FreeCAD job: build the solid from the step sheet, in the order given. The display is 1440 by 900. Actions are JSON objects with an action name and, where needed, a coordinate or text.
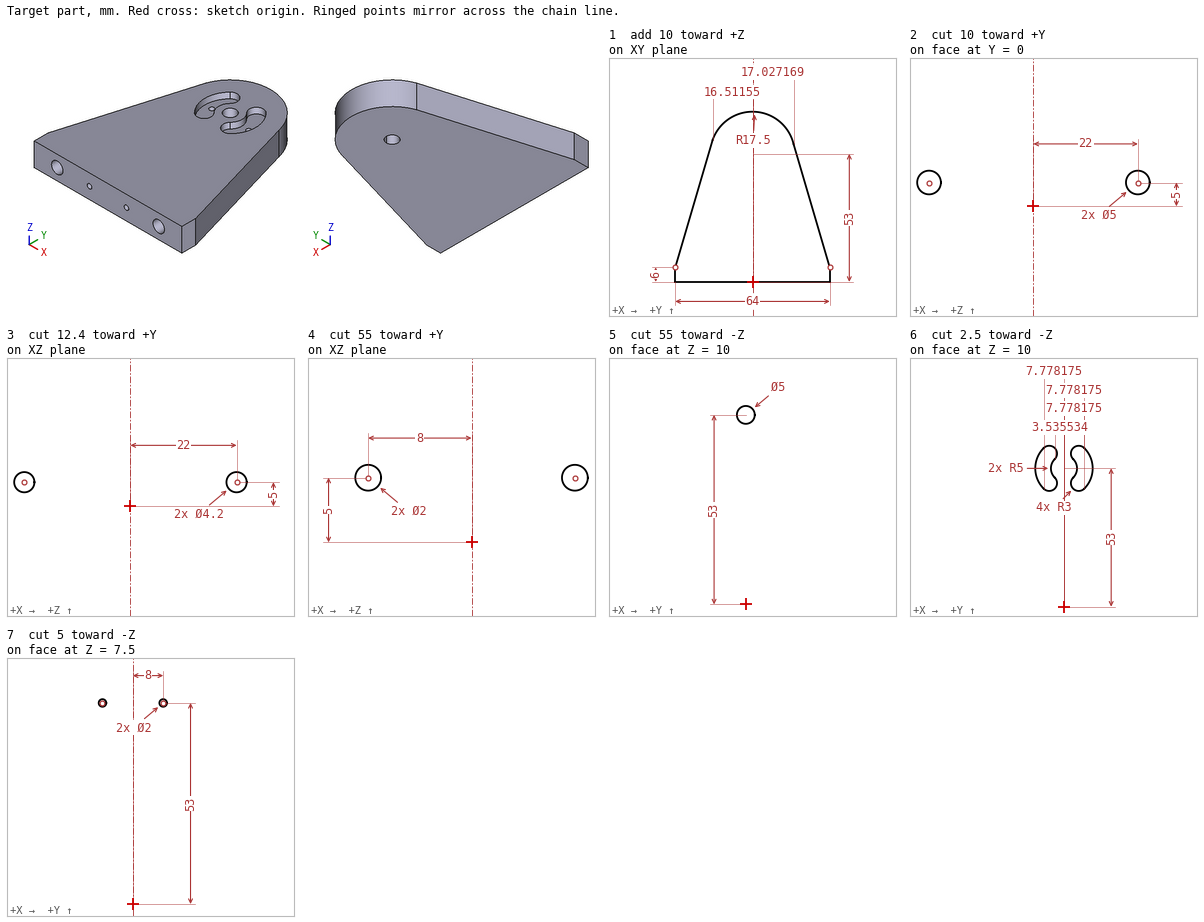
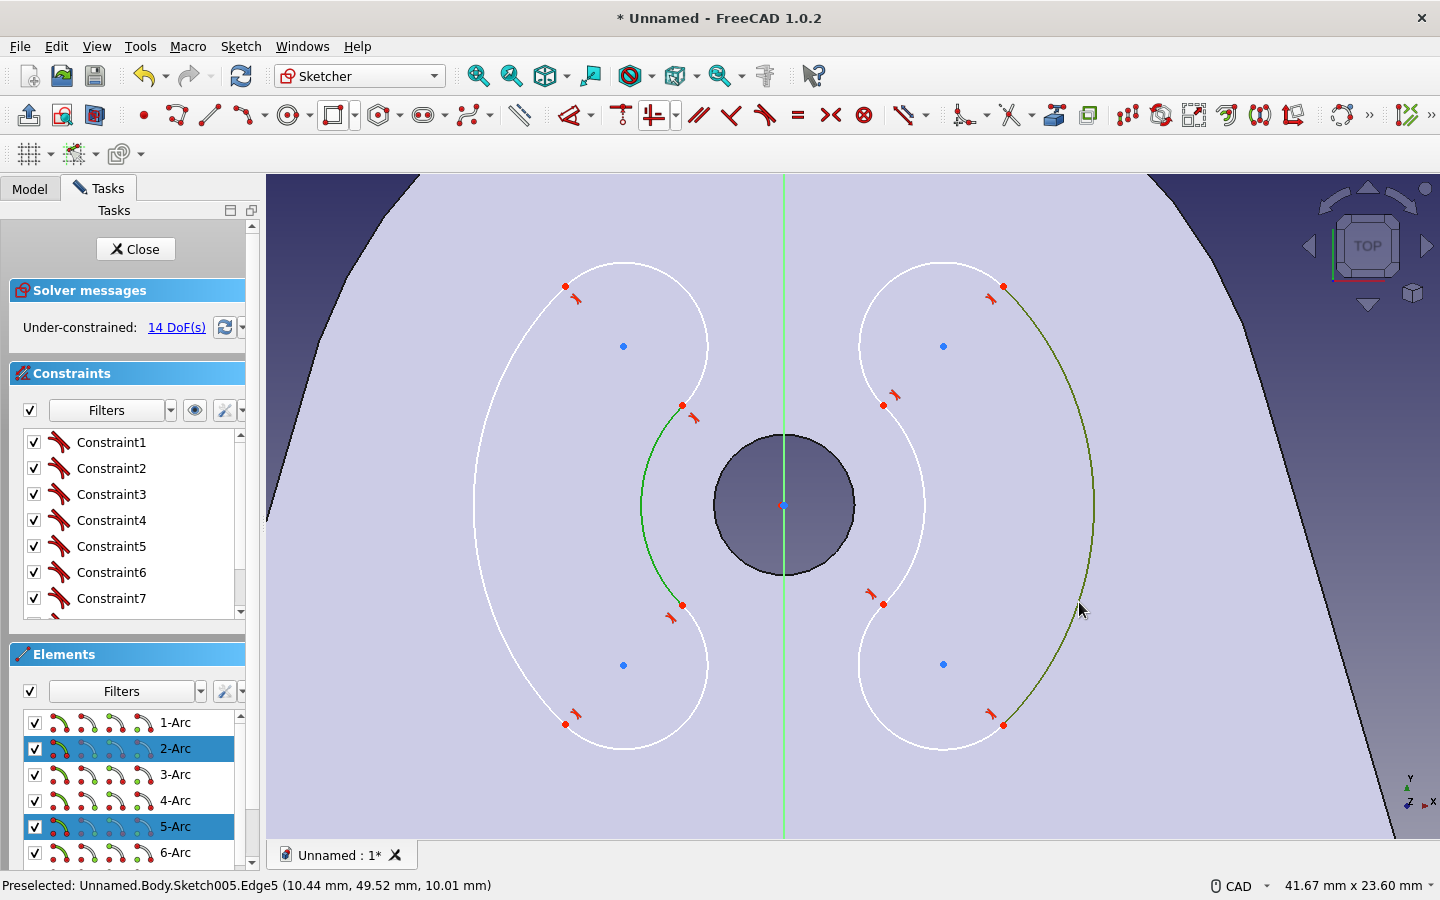
{"action": "left_click", "coordinate": [621, 116]}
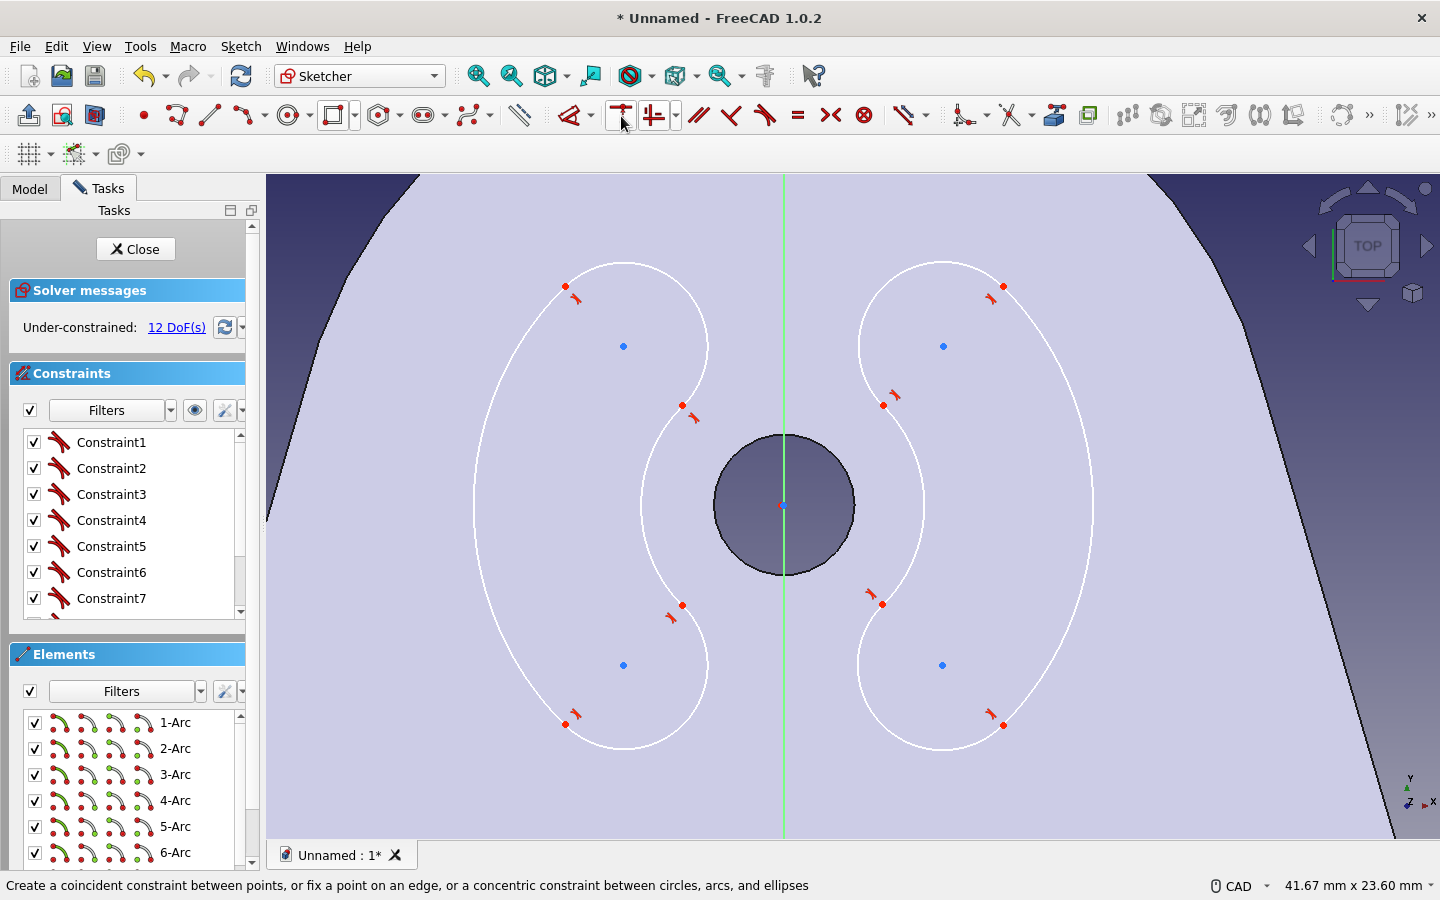
{"action": "left_click", "coordinate": [648, 462]}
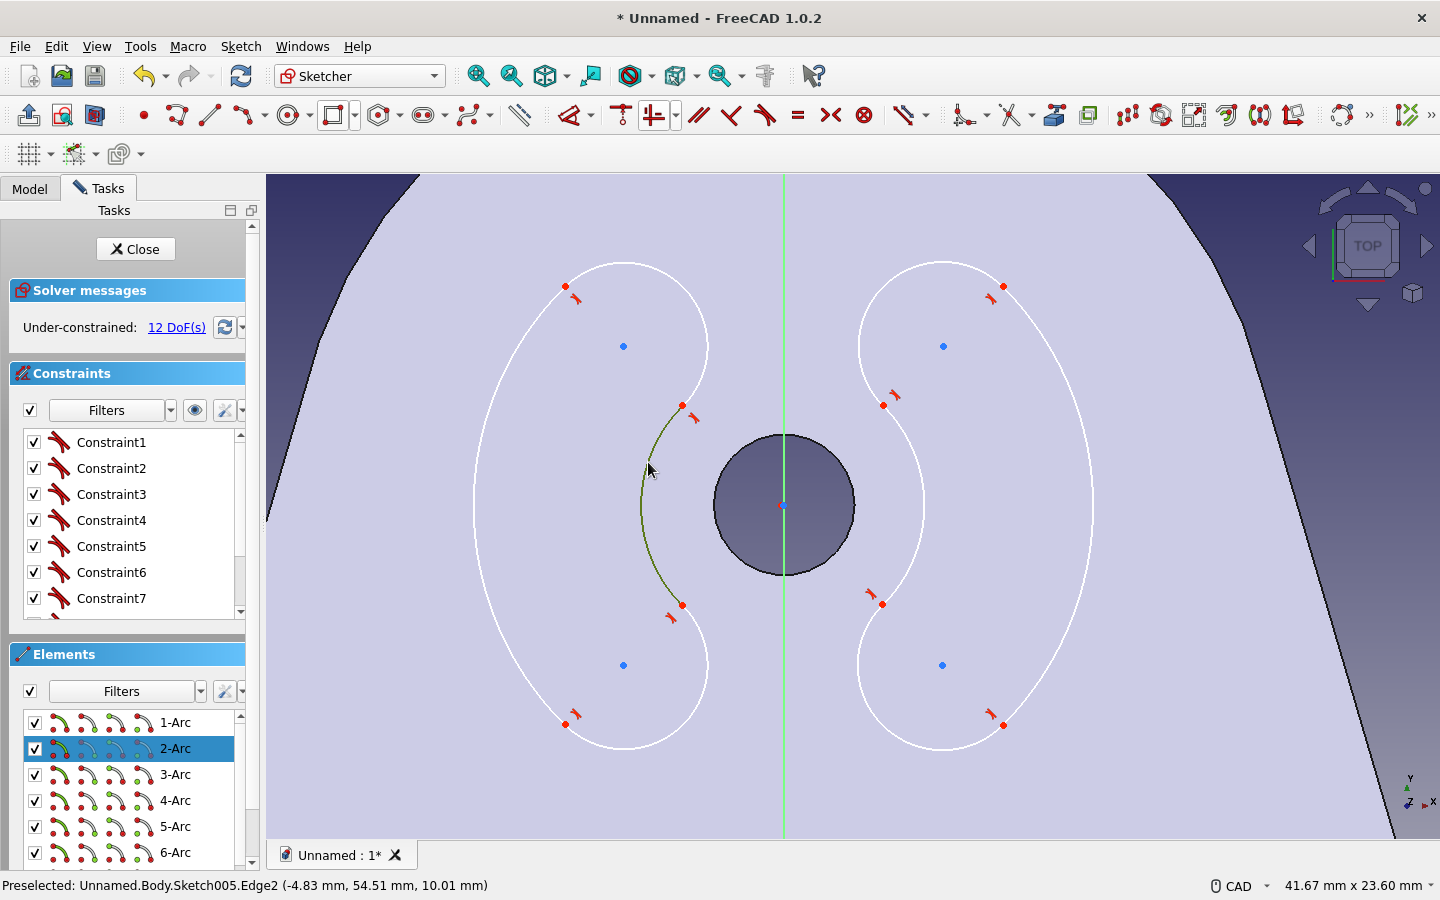
{"action": "left_click", "coordinate": [917, 549]}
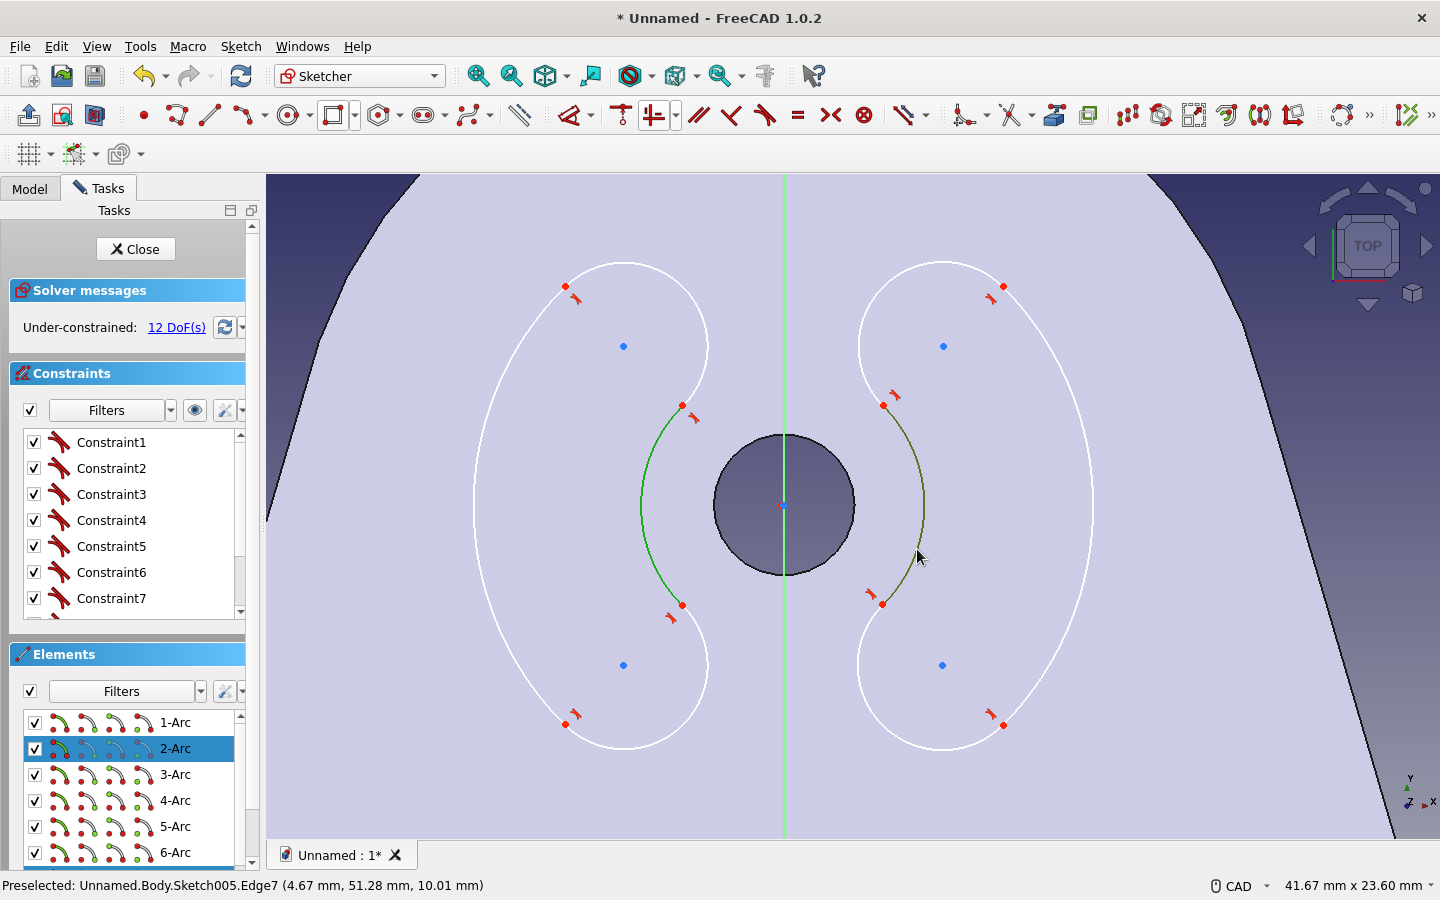
{"action": "left_click", "coordinate": [621, 116]}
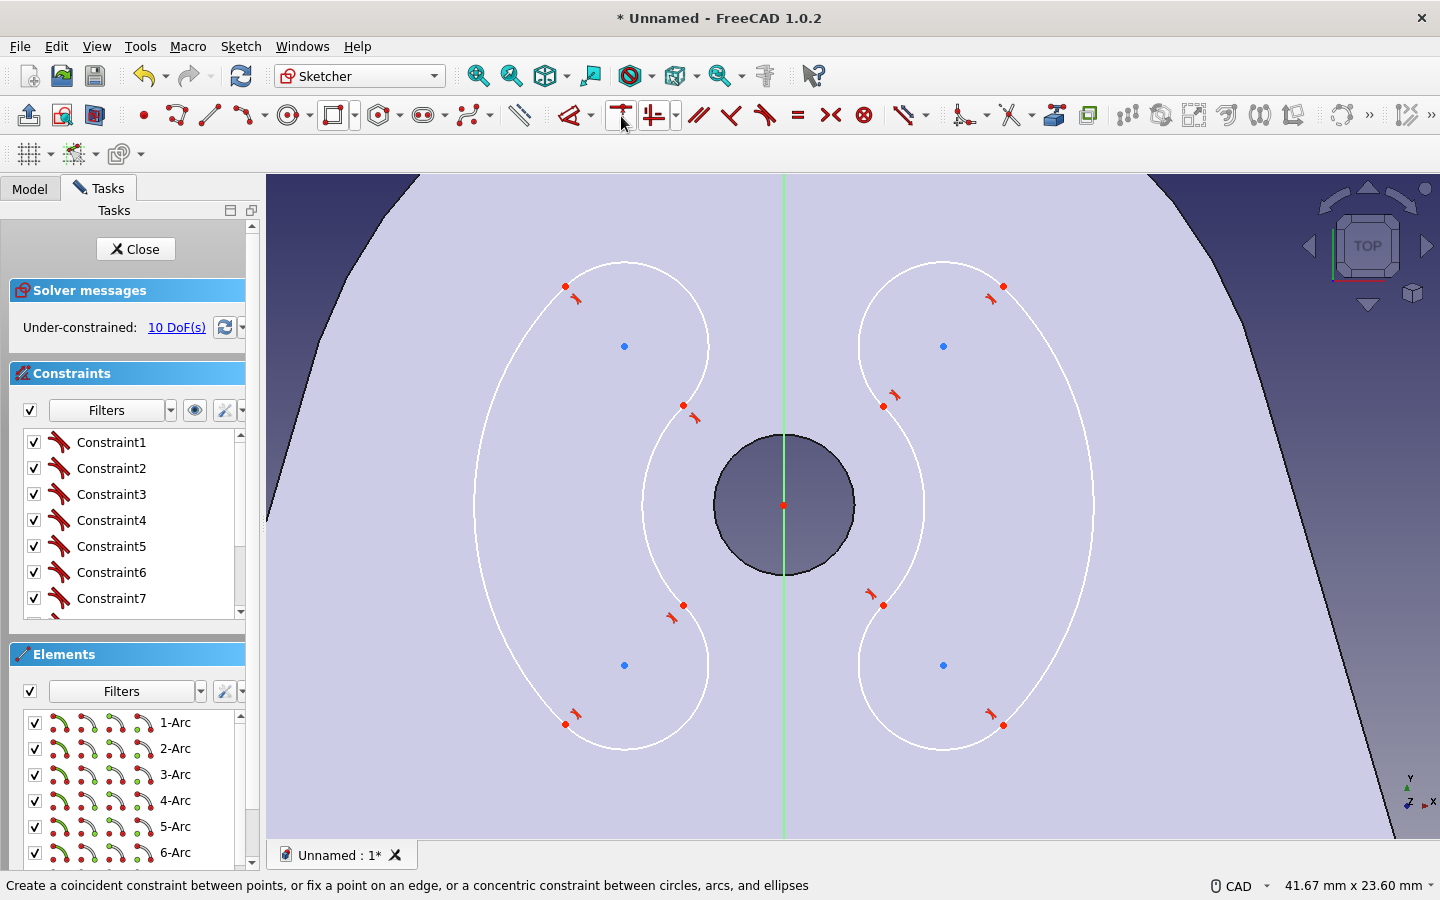
{"action": "left_click", "coordinate": [489, 410]}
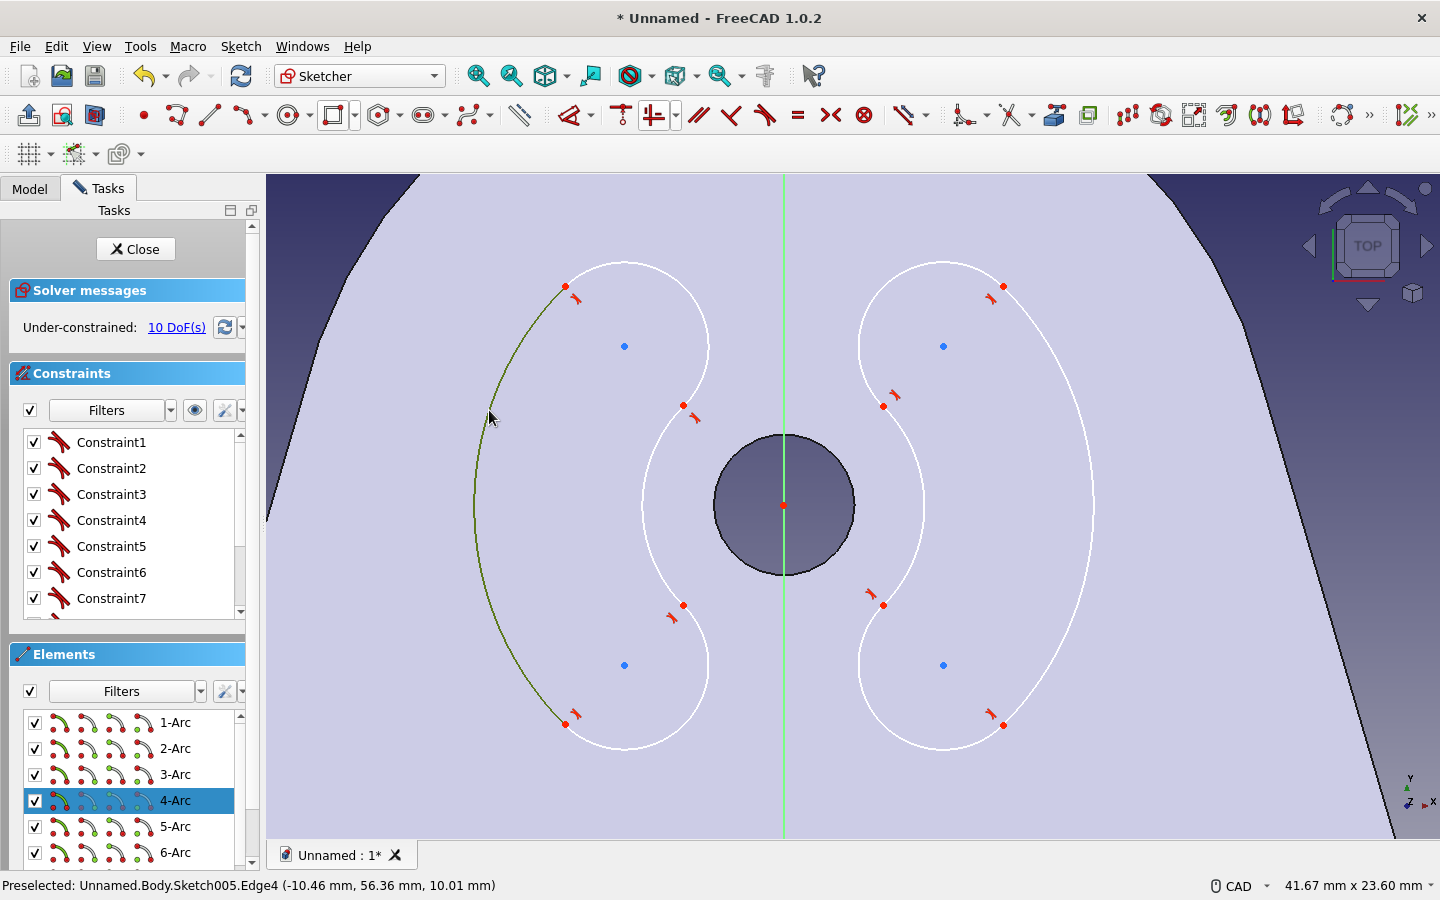
{"action": "left_click", "coordinate": [1078, 602]}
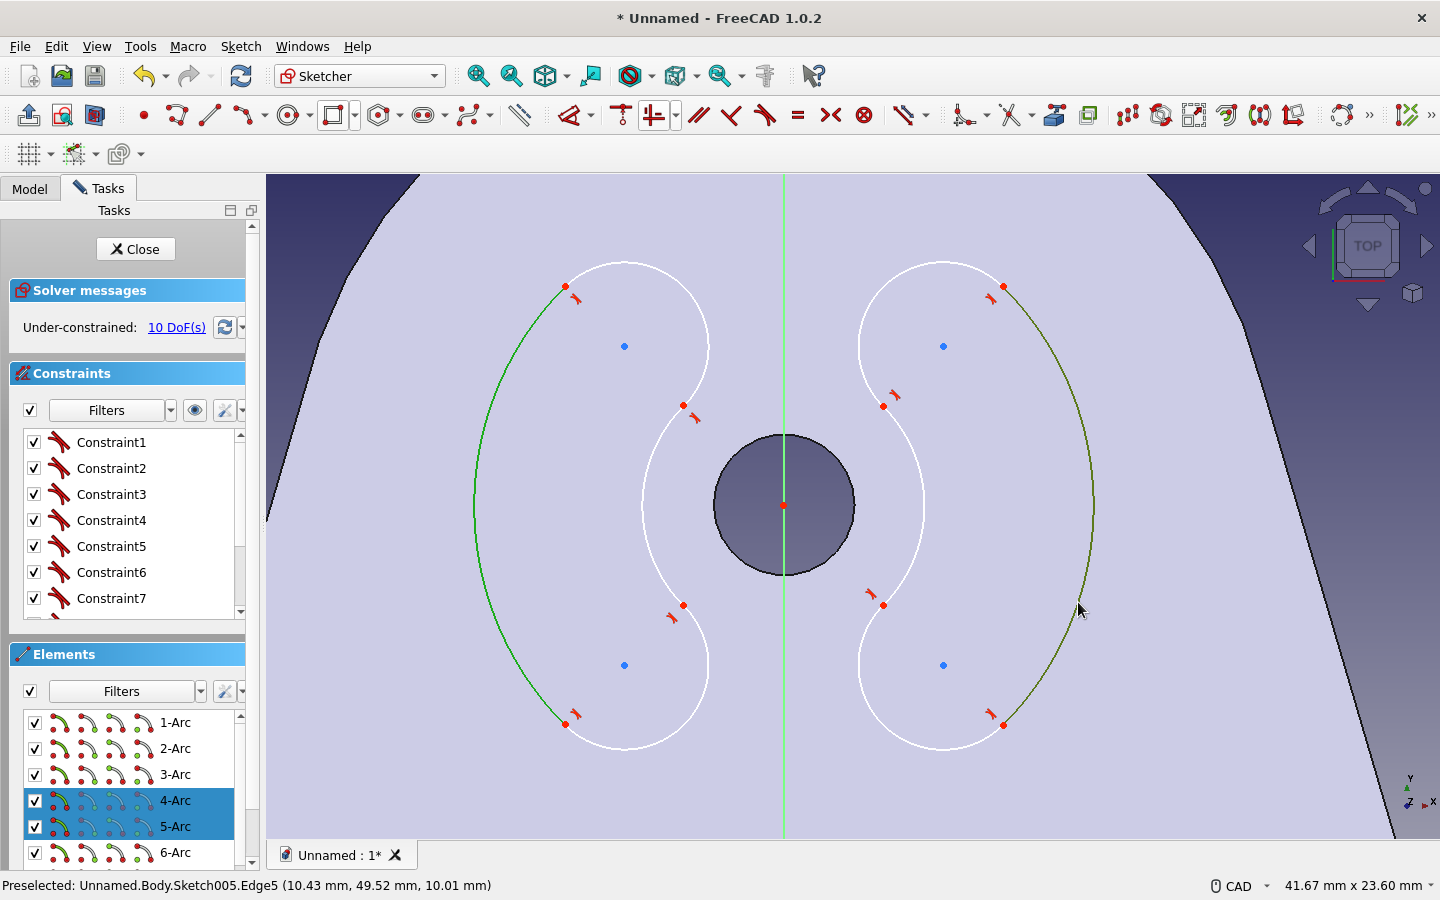
{"action": "key", "text": "e"}